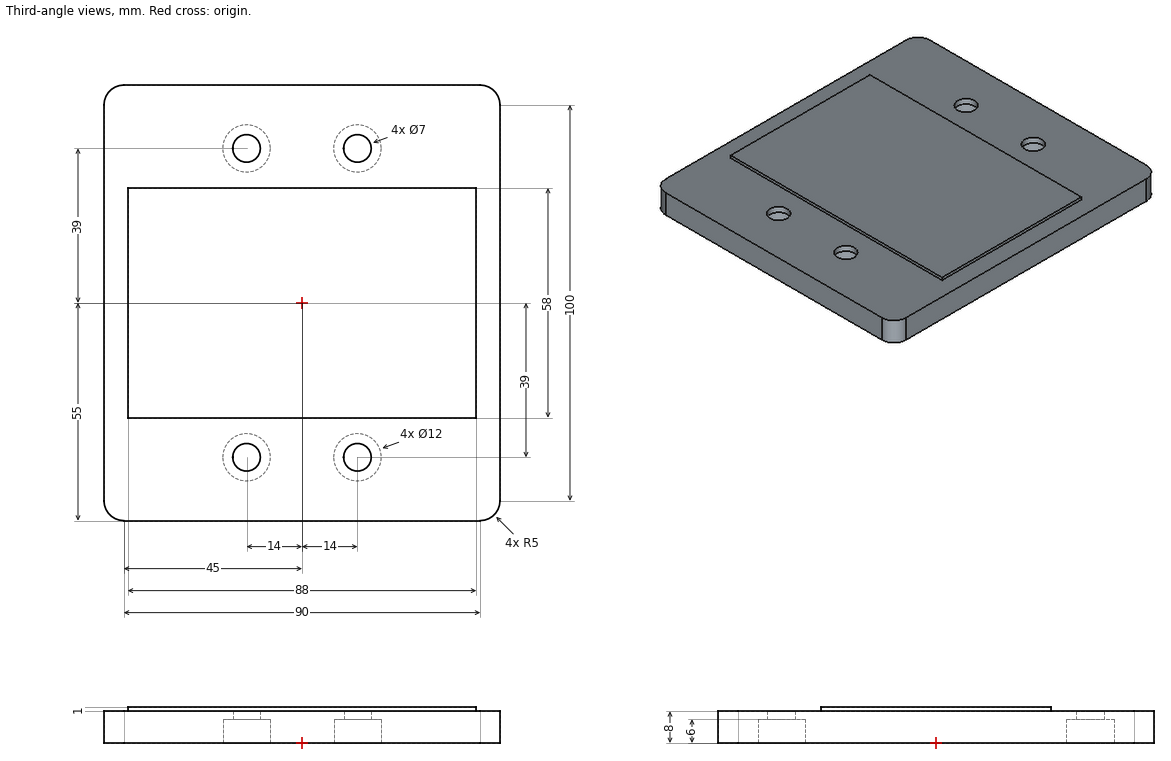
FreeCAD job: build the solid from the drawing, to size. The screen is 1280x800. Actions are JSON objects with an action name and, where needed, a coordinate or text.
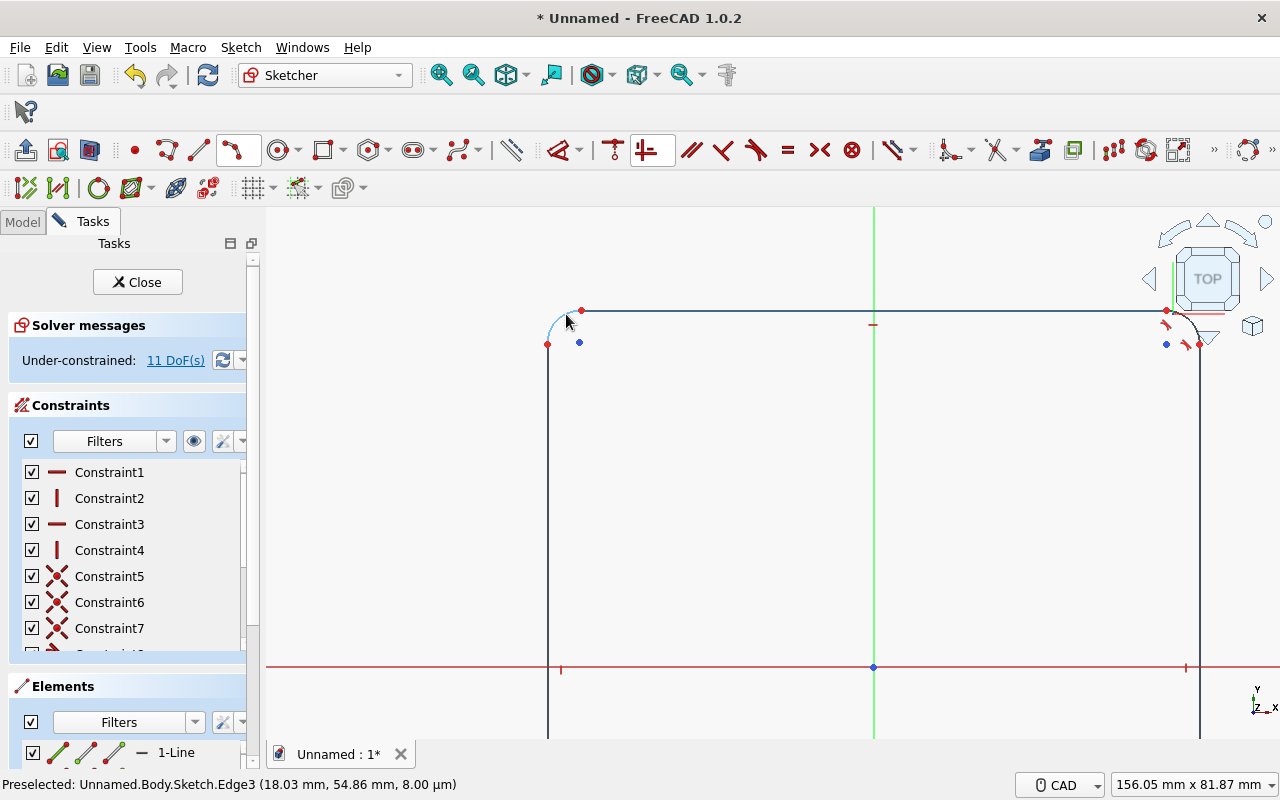
{"action": "left_click", "coordinate": [566, 314]}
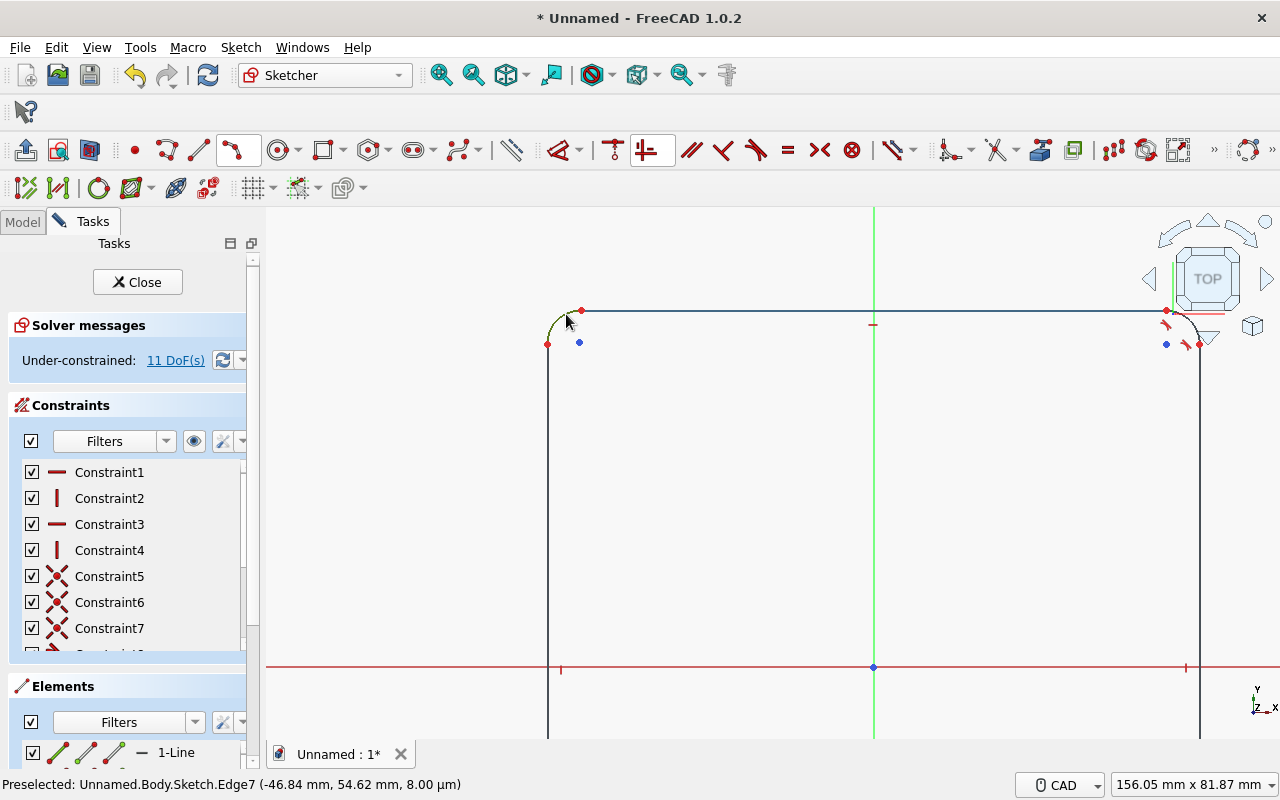
{"action": "left_click", "coordinate": [756, 150]}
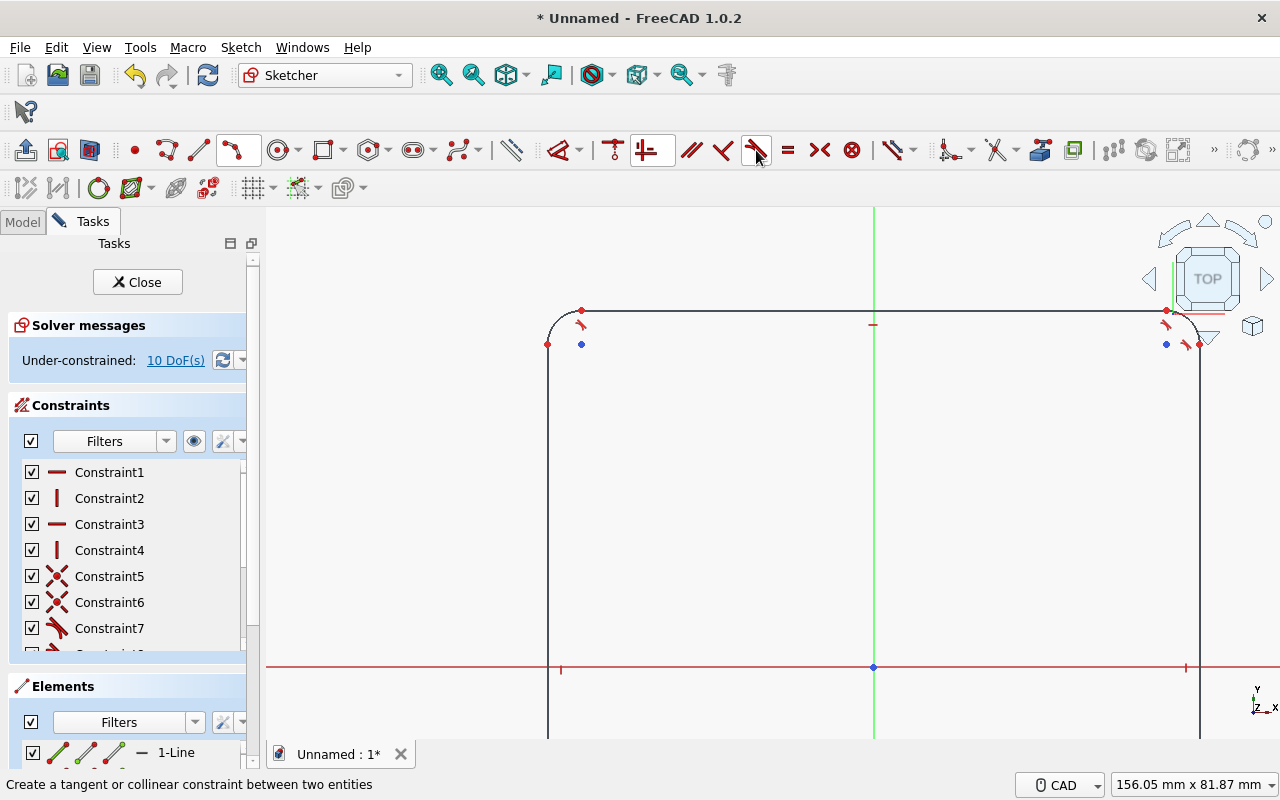
{"action": "left_click", "coordinate": [548, 539]}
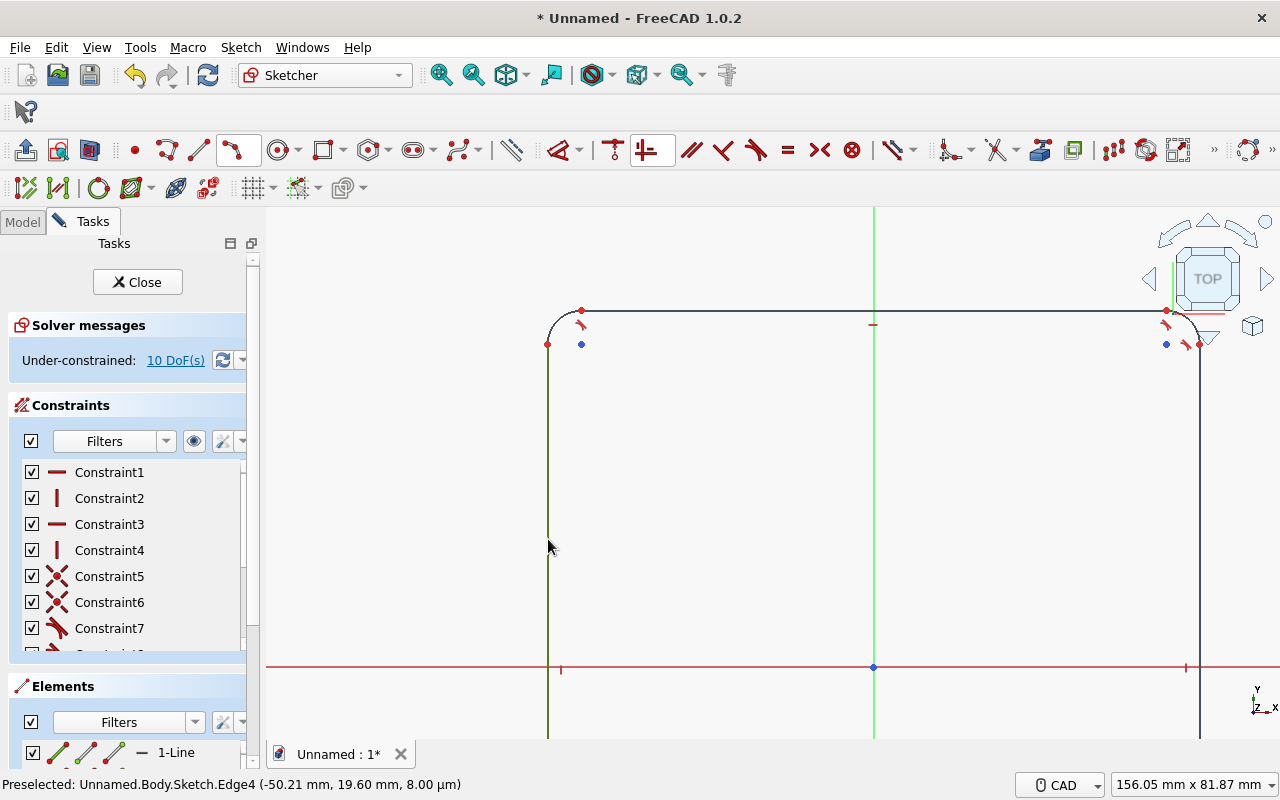
{"action": "left_click", "coordinate": [566, 314]}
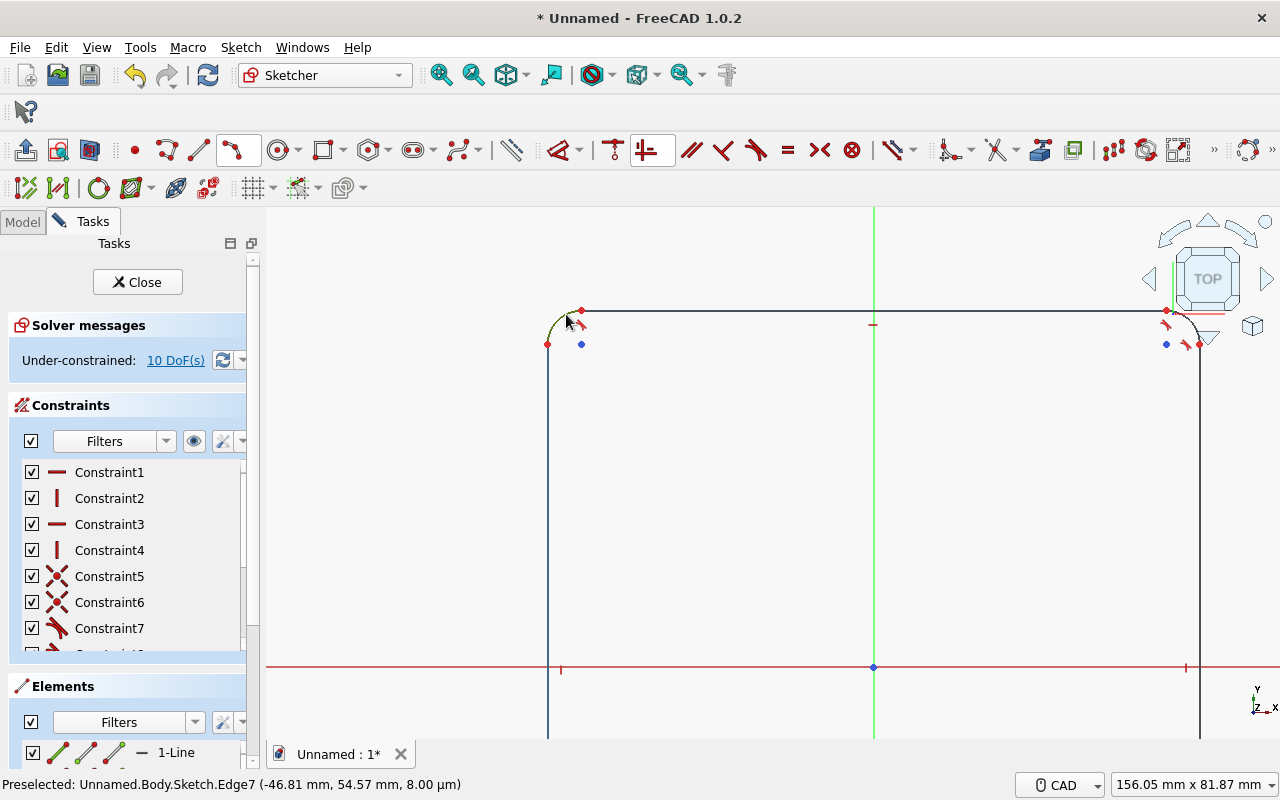
{"action": "key", "text": "t"}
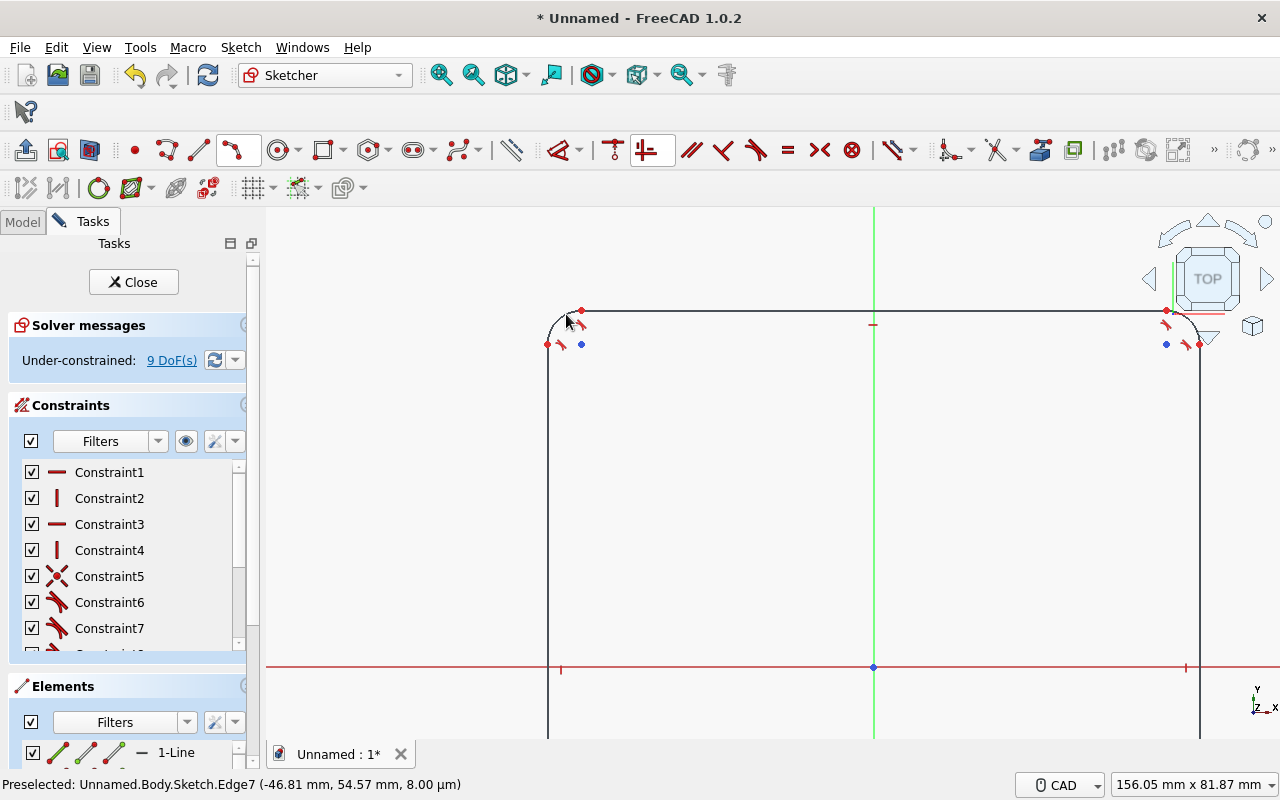
{"action": "left_click", "coordinate": [548, 539]}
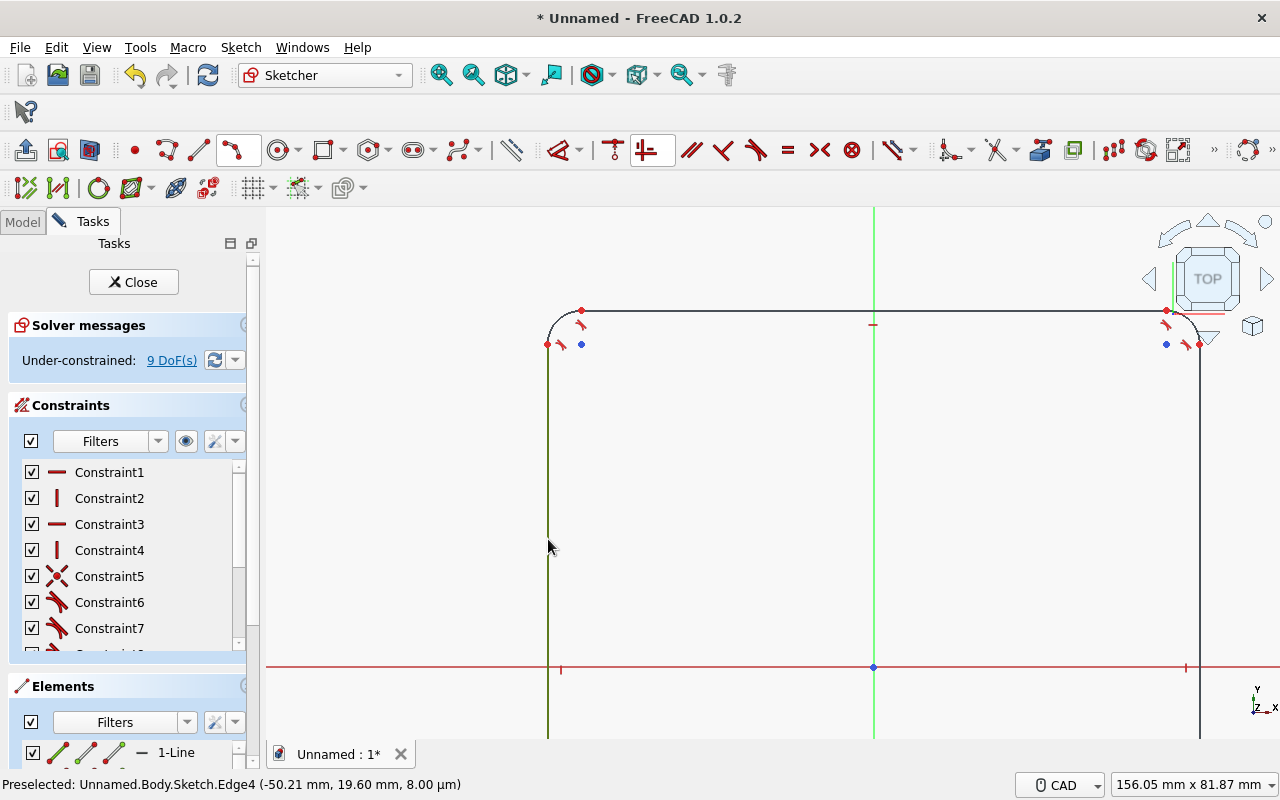
{"action": "scroll", "coordinate": [566, 314], "scroll_direction": "down", "scroll_amount": 4}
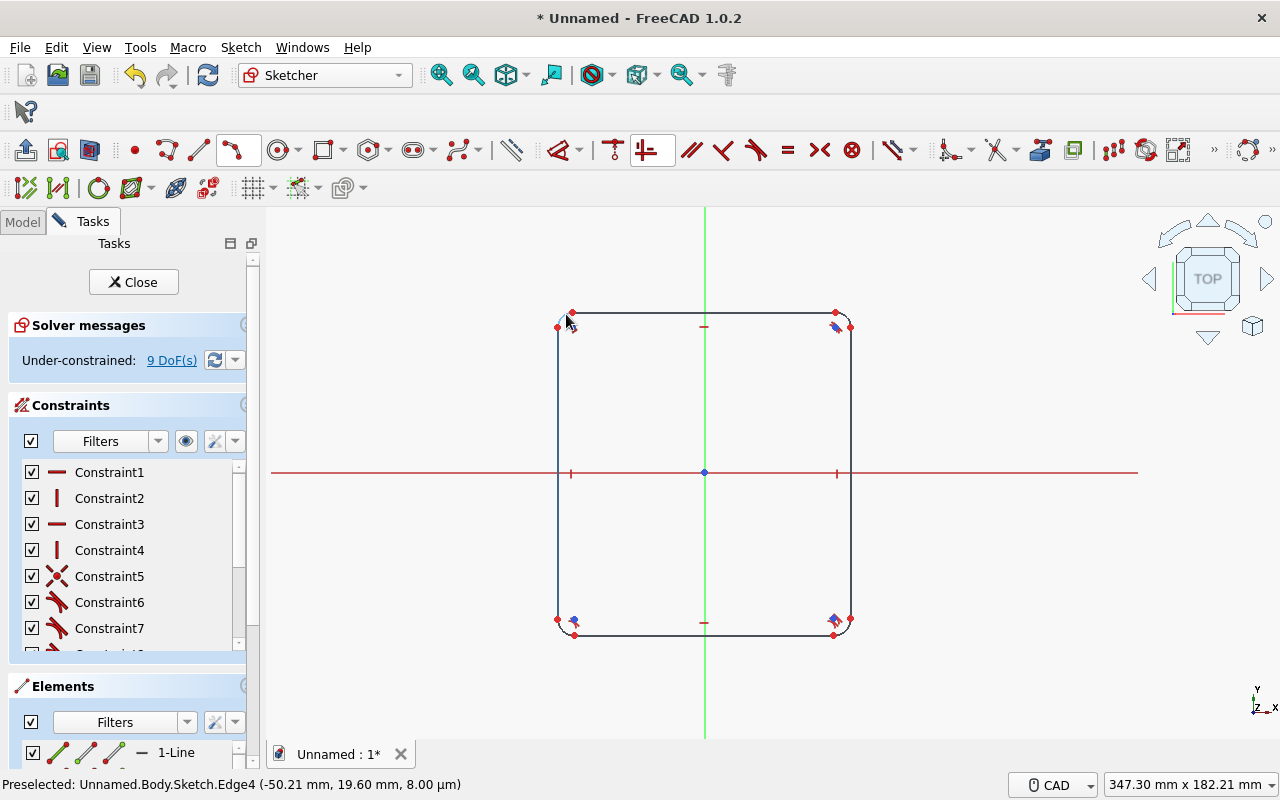
{"action": "scroll", "coordinate": [560, 627], "scroll_direction": "up", "scroll_amount": 3}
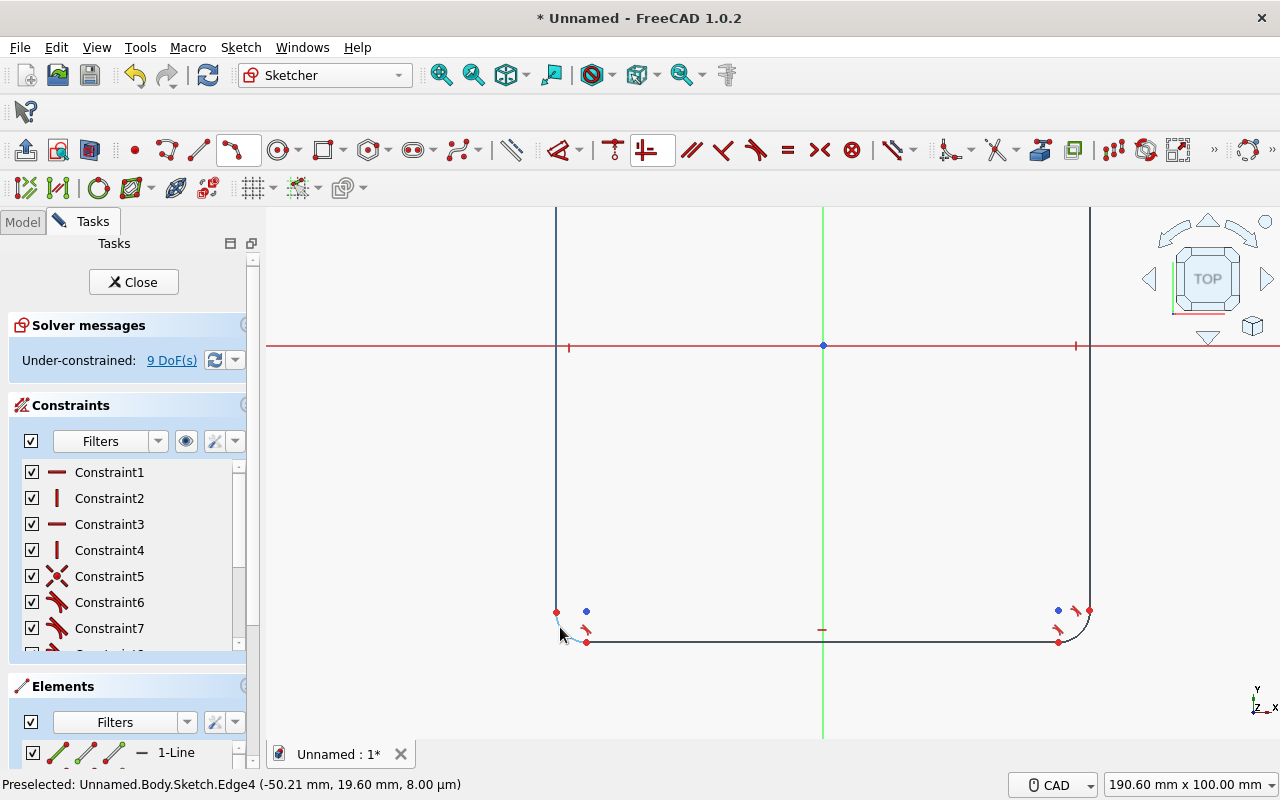
{"action": "left_click", "coordinate": [560, 626]}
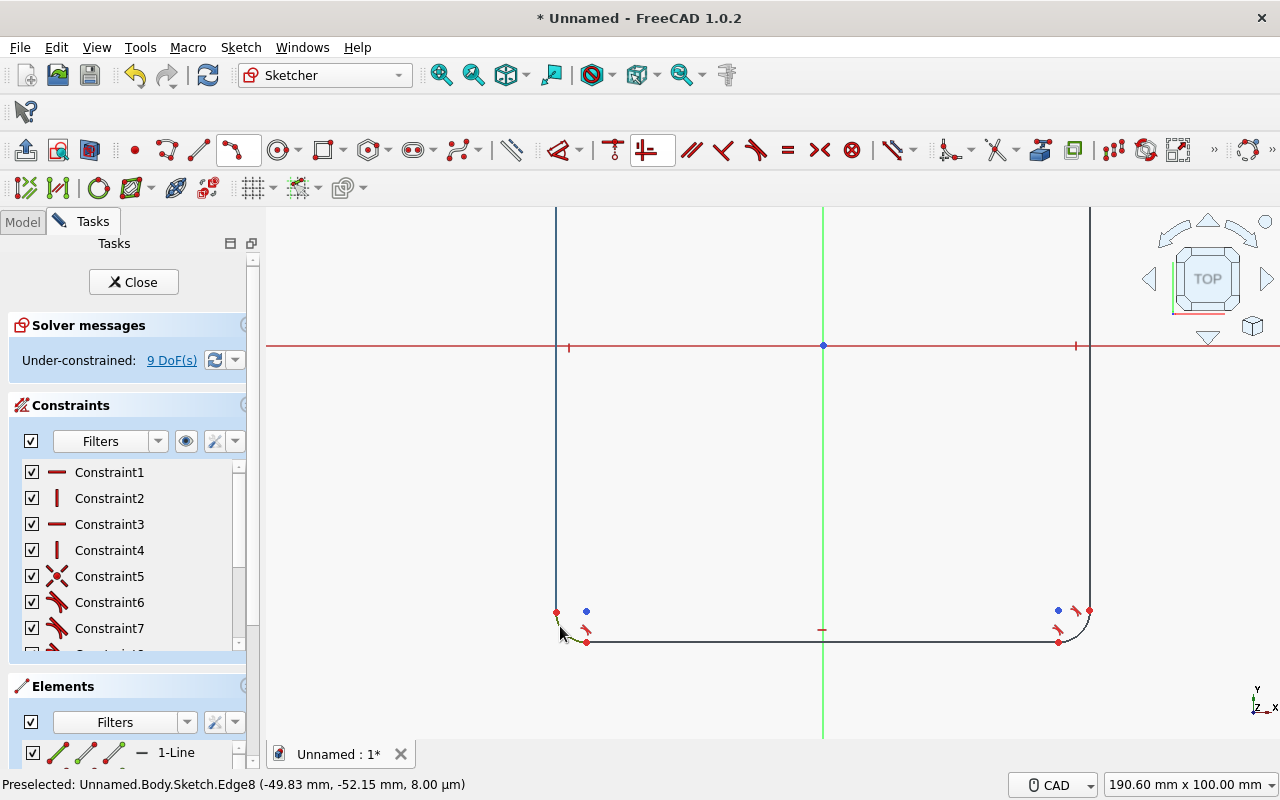
{"action": "key", "text": "t"}